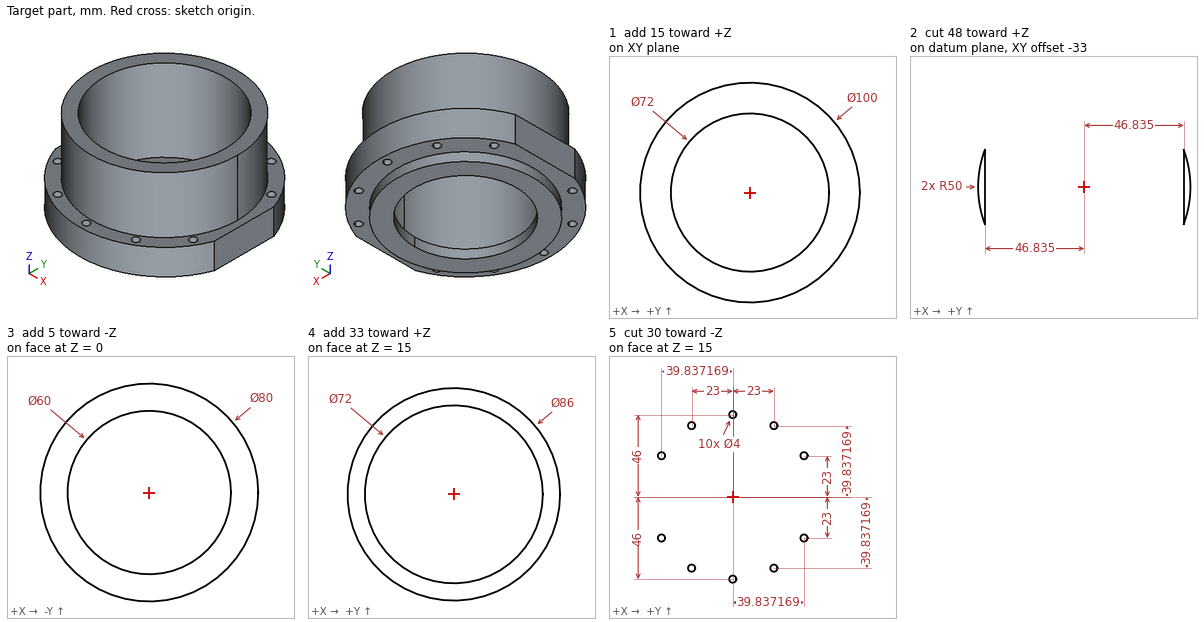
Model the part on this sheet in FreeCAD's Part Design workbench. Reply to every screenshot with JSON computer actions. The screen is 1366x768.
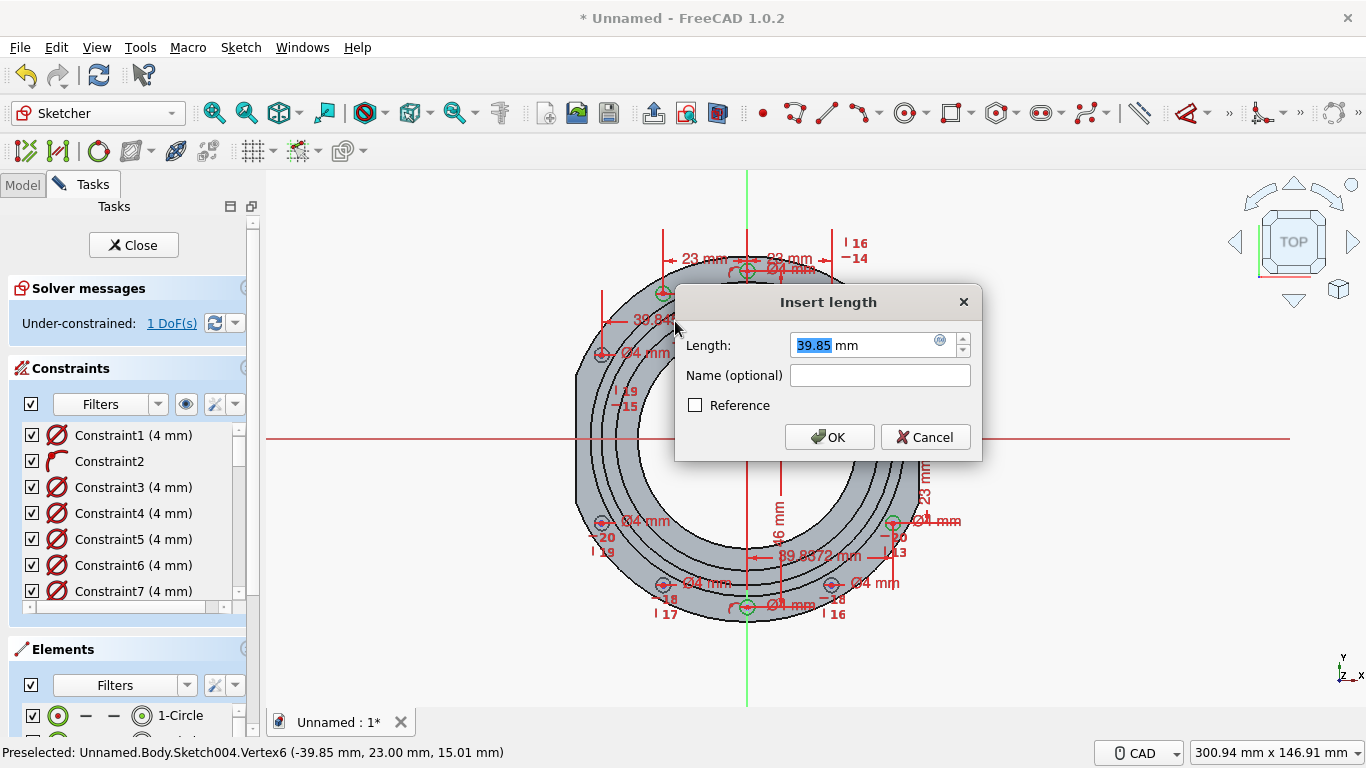
{"action": "type", "text": "39.837169"}
{"action": "key", "text": "Return"}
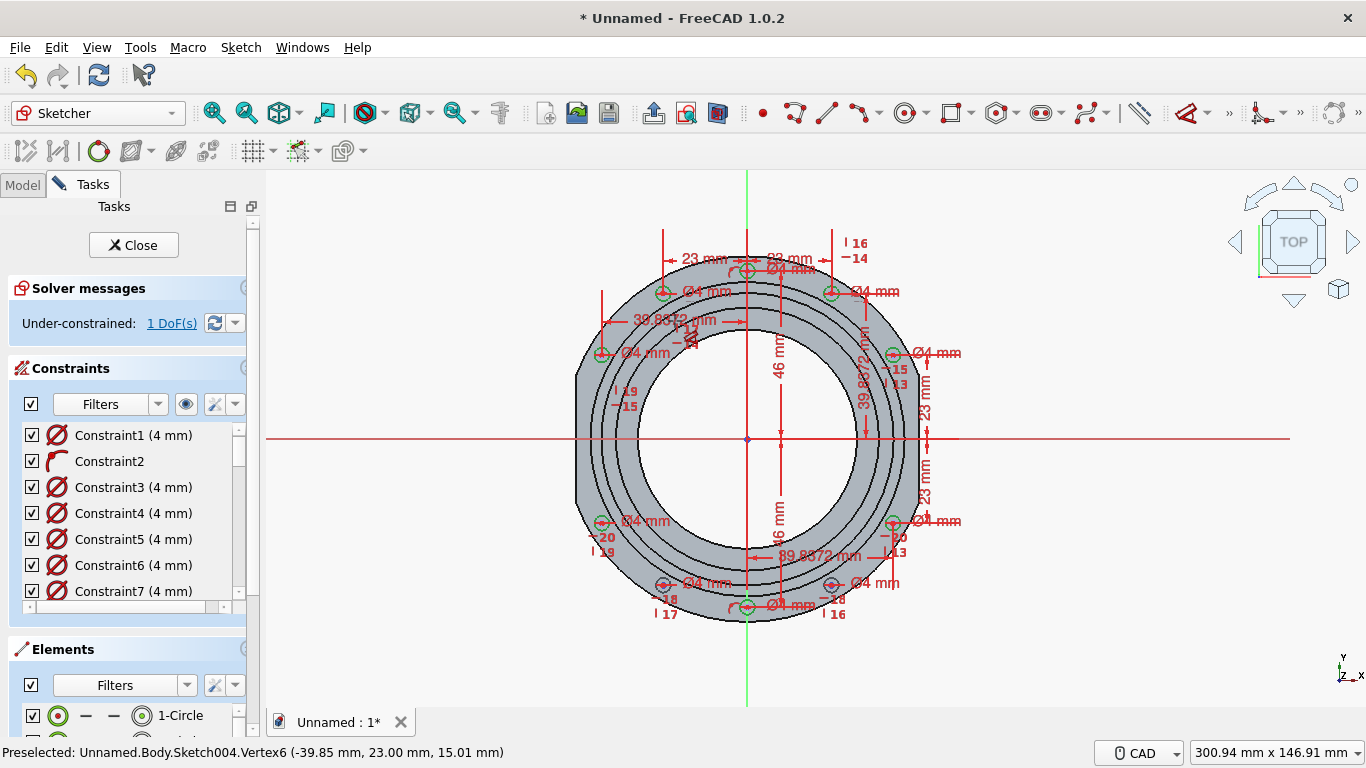
{"action": "left_click", "coordinate": [832, 585]}
{"action": "left_click", "coordinate": [866, 512]}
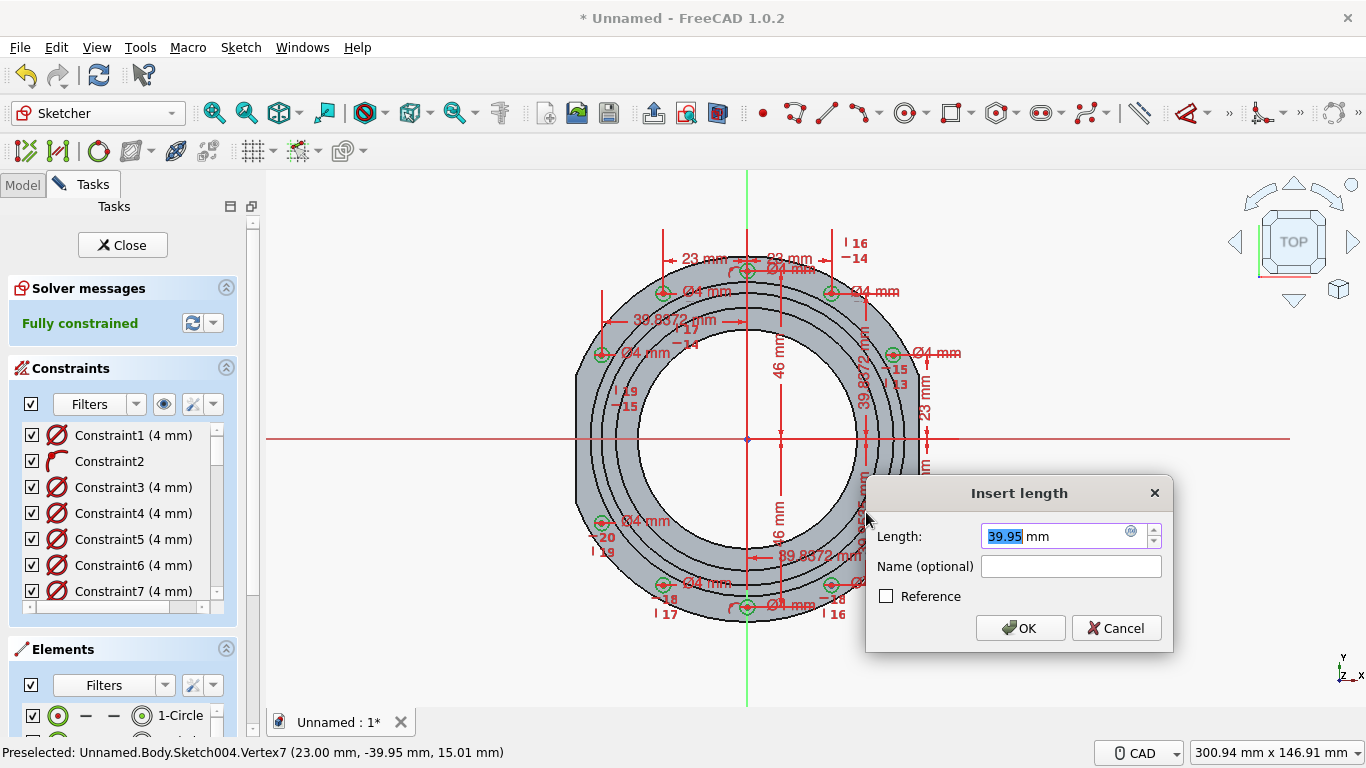
{"action": "type", "text": "39.837169"}
{"action": "key", "text": "Return"}
{"action": "key", "text": "Escape"}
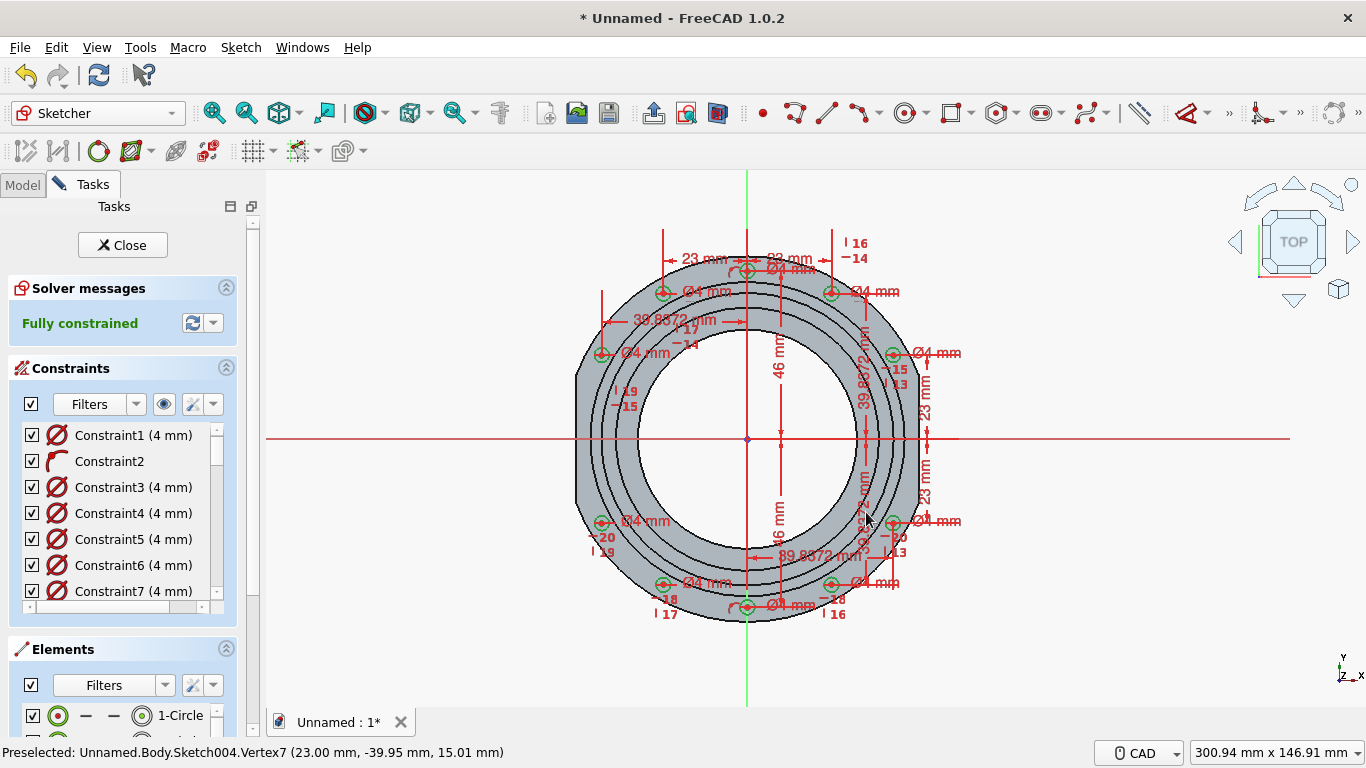
{"action": "left_click", "coordinate": [123, 245]}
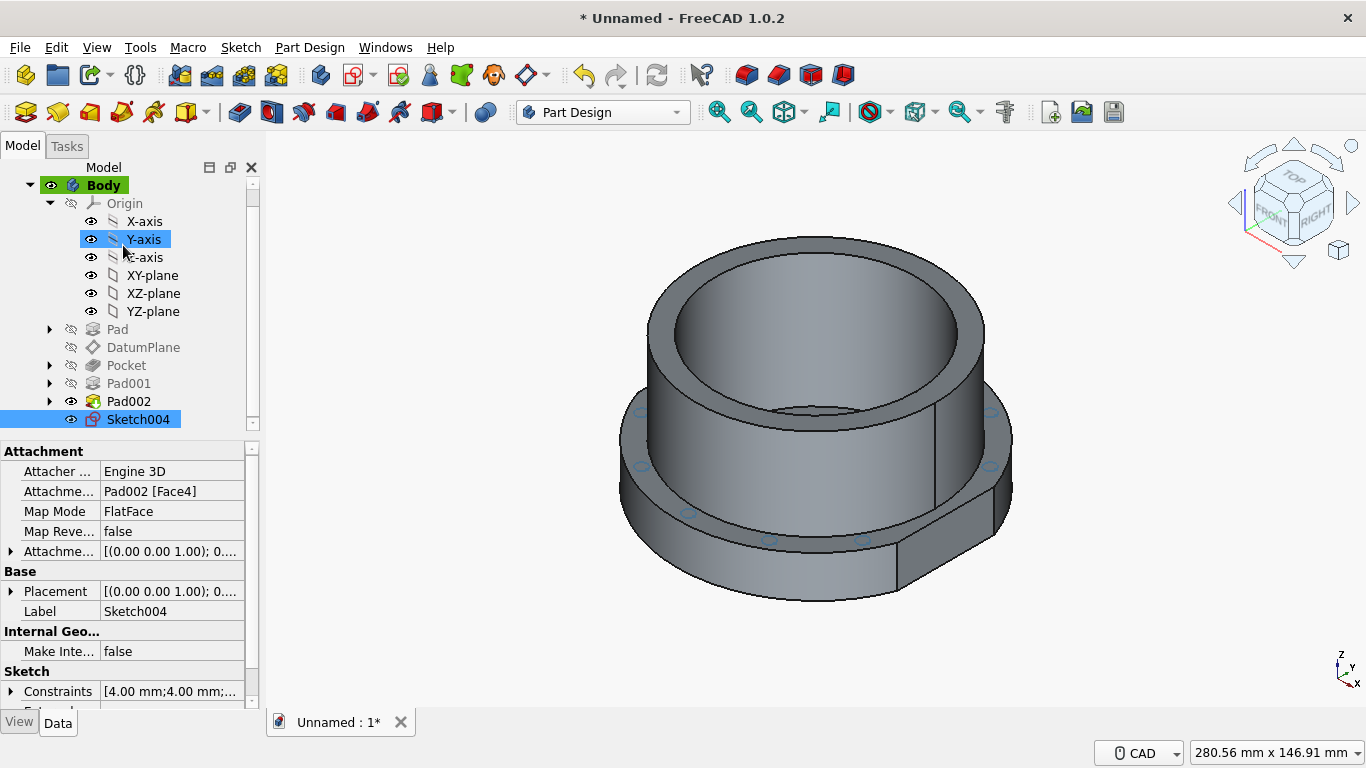
{"action": "left_click", "coordinate": [240, 112]}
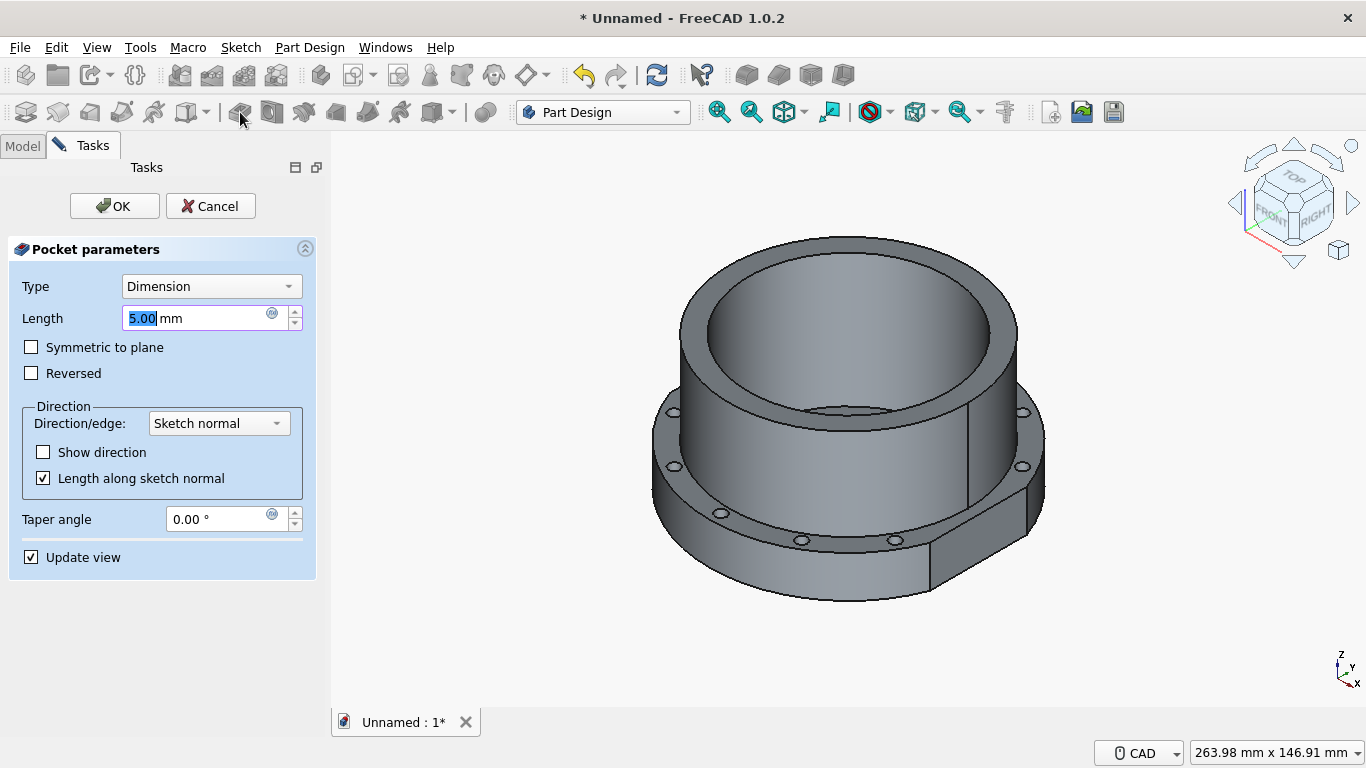
{"action": "type", "text": "30"}
{"action": "key", "text": "Tab"}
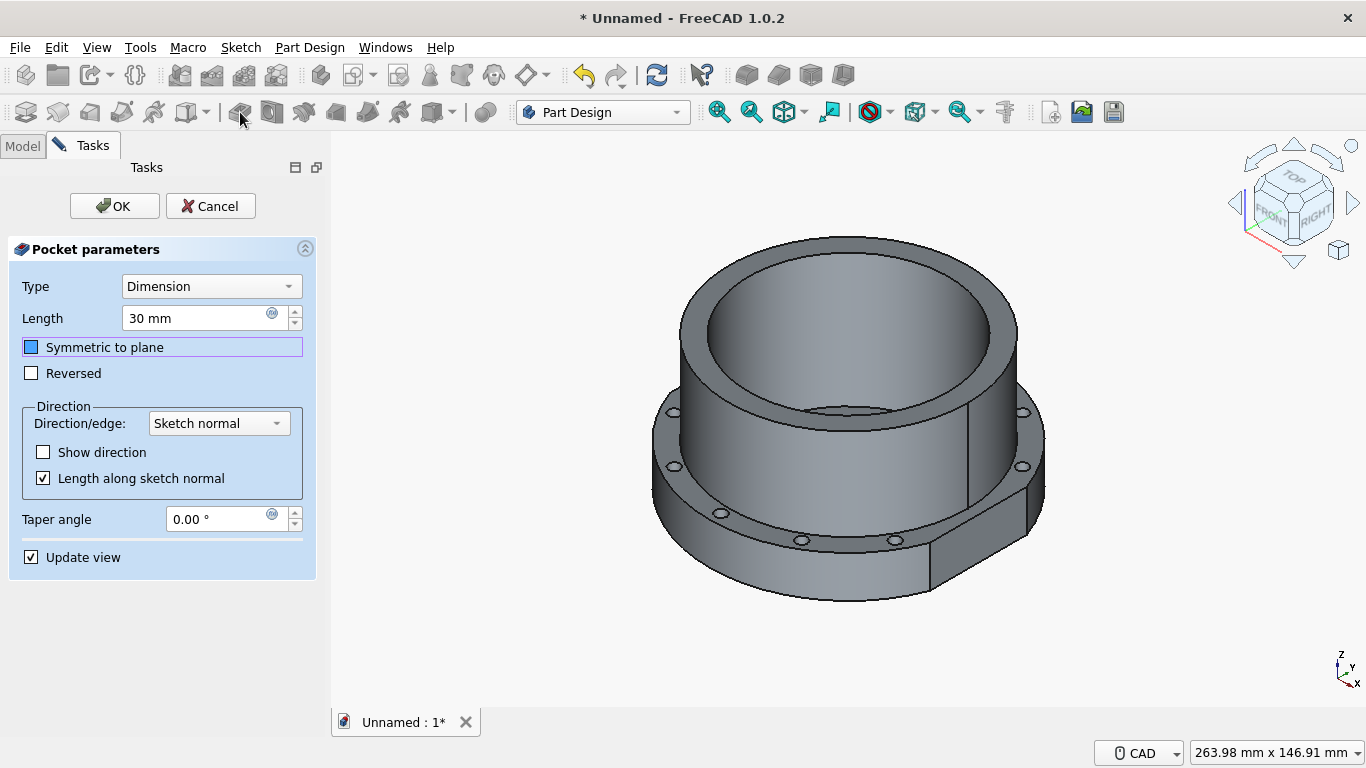
{"action": "left_click", "coordinate": [115, 206]}